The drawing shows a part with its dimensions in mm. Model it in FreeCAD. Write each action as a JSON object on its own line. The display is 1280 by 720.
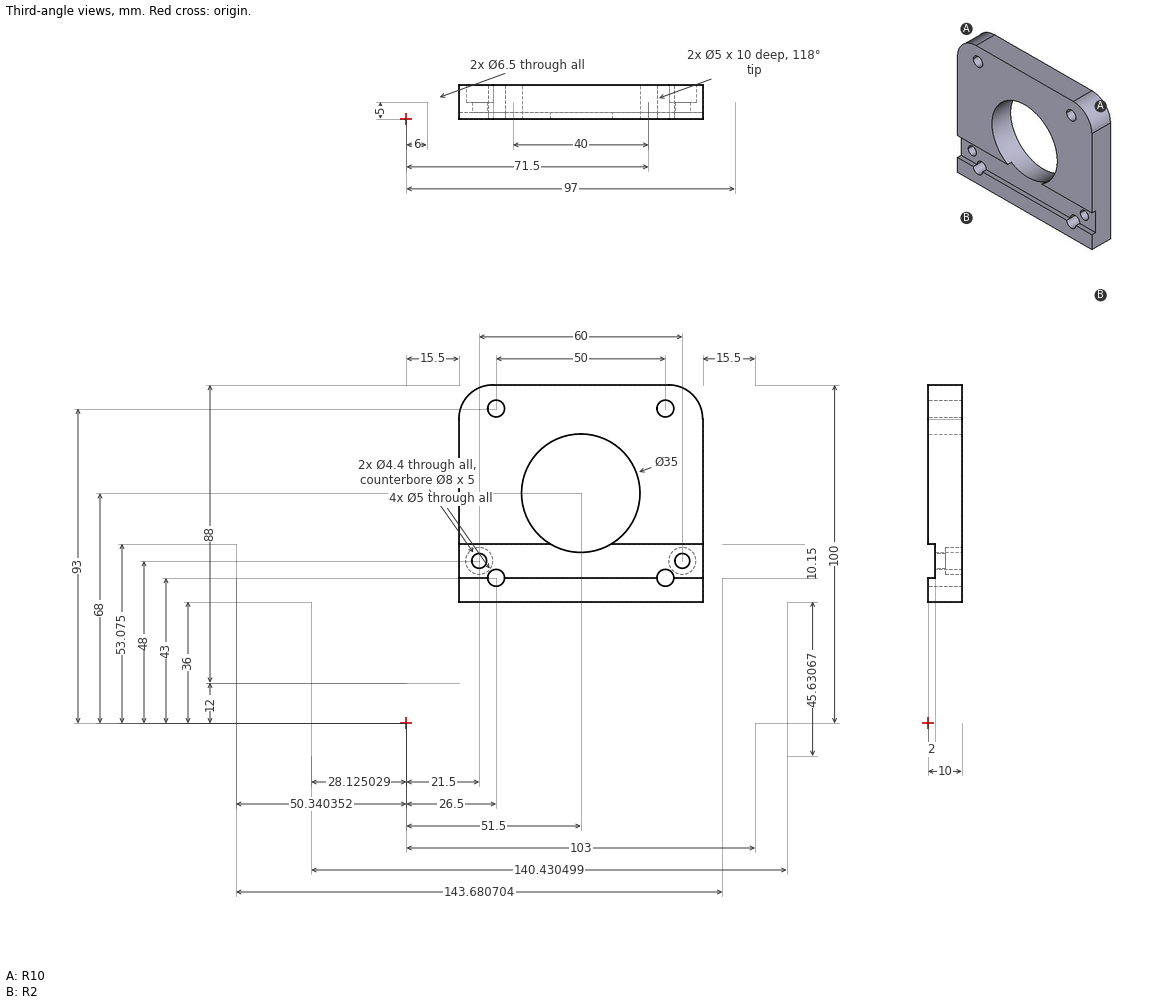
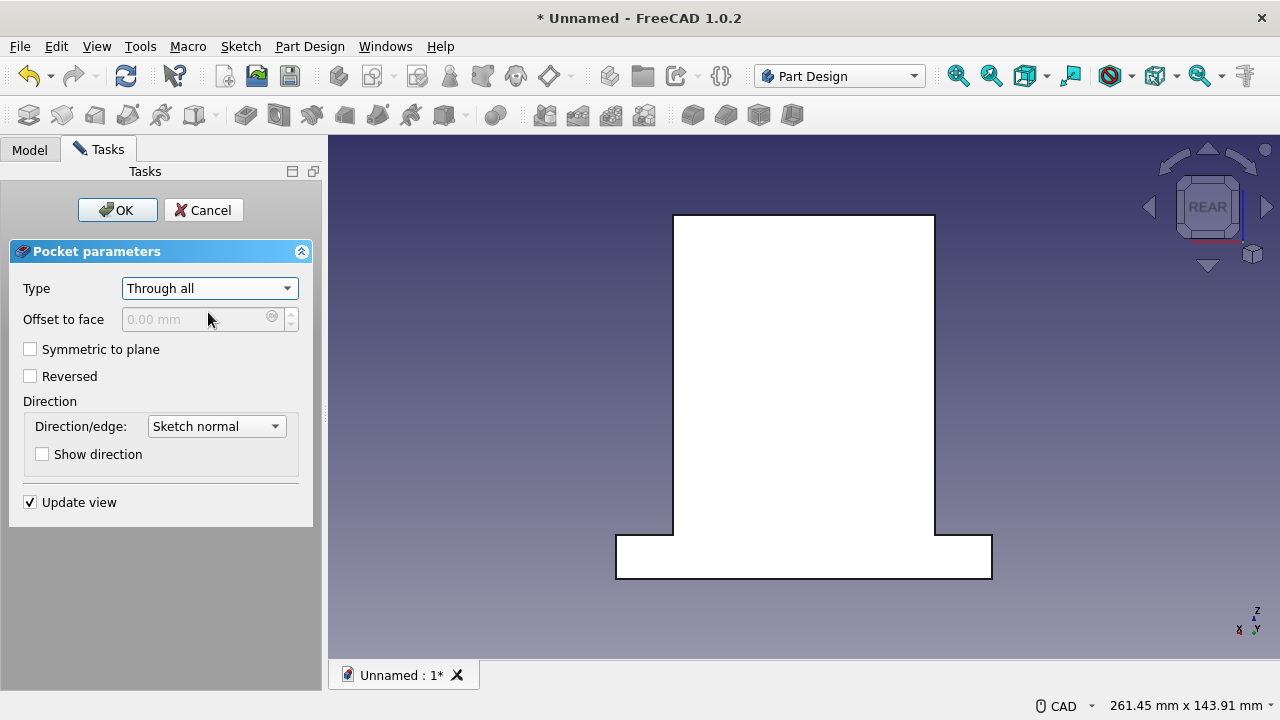
{"action": "left_click", "coordinate": [118, 210]}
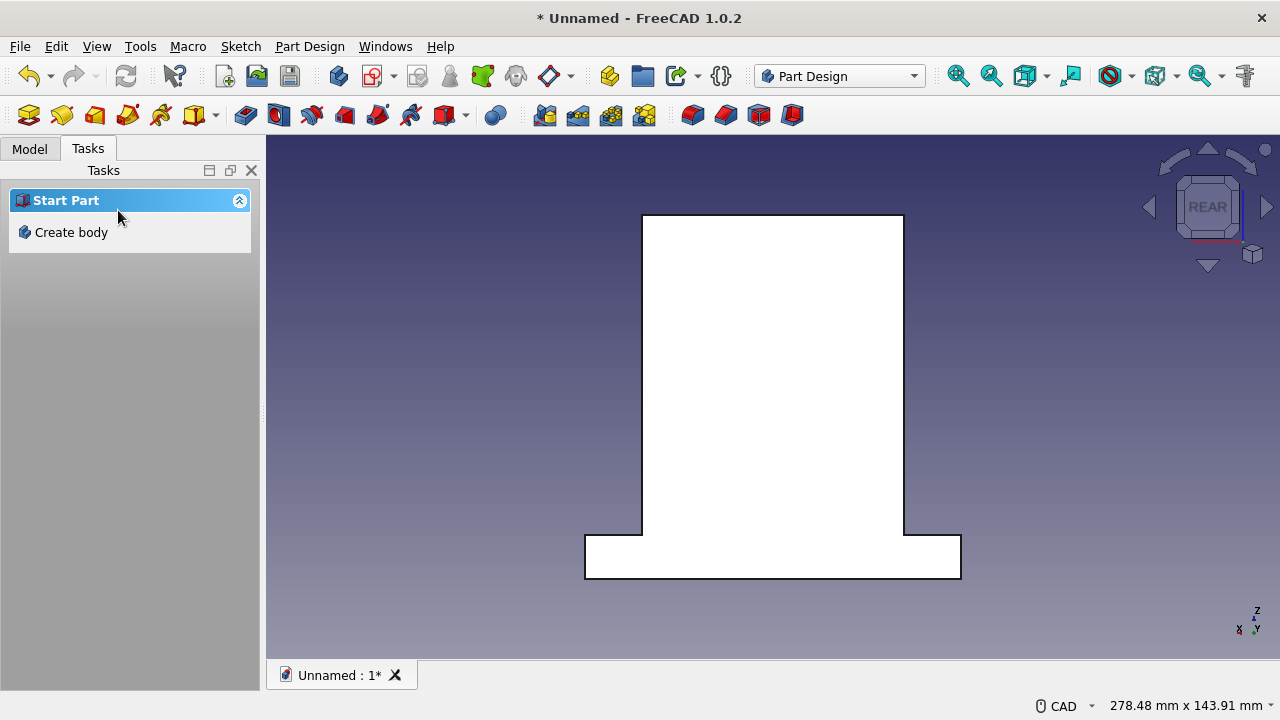
{"action": "key", "text": "0"}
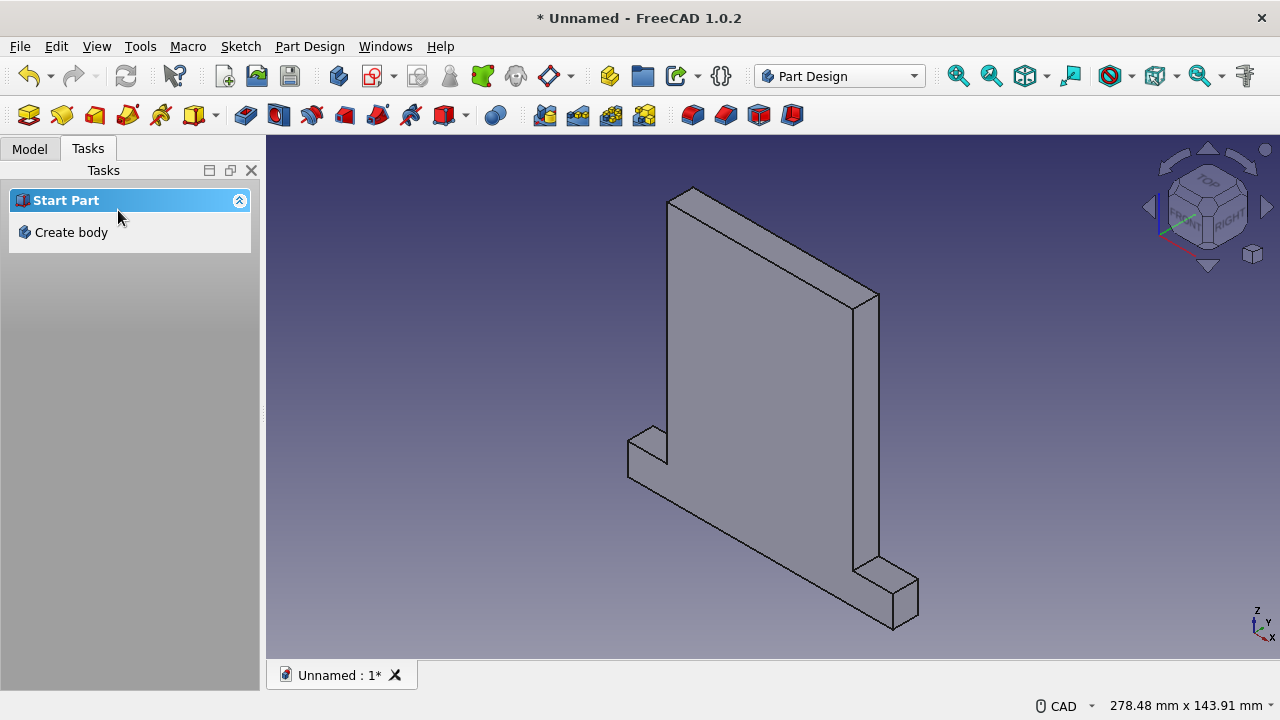
{"action": "left_click", "coordinate": [655, 441]}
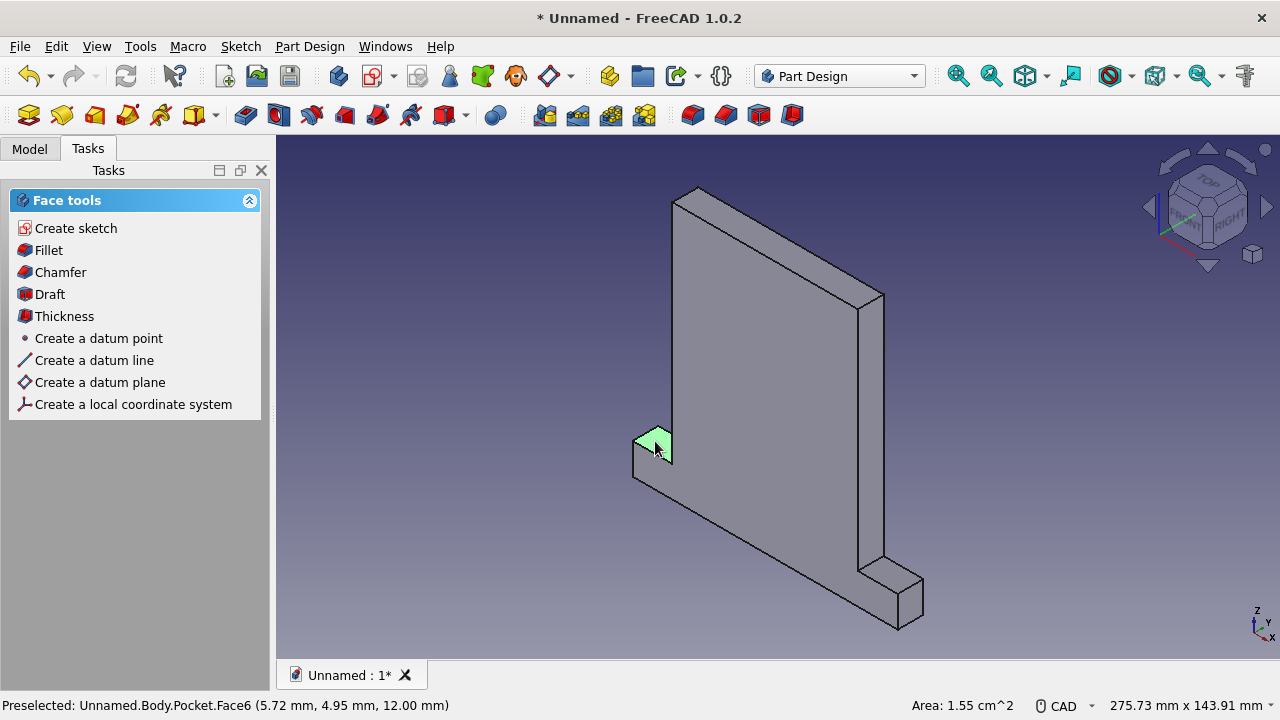
{"action": "left_click", "coordinate": [372, 76]}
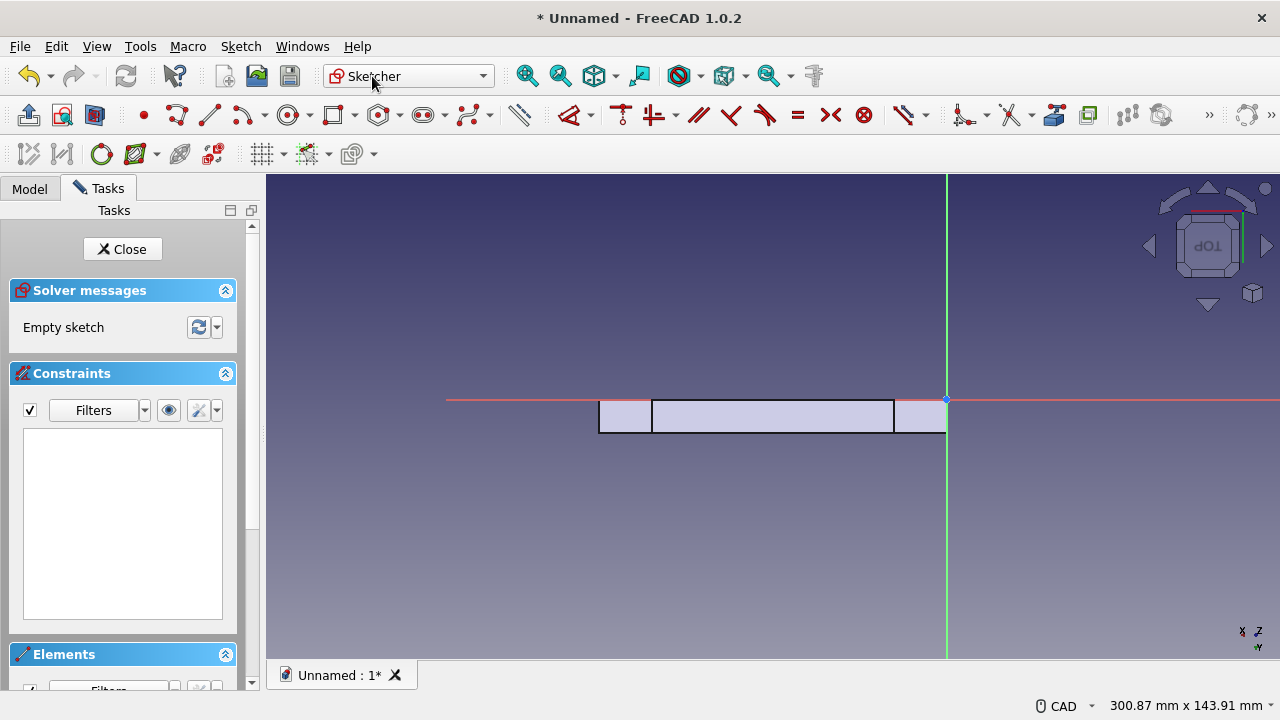
{"action": "scroll", "coordinate": [867, 410], "scroll_direction": "up", "scroll_amount": 3}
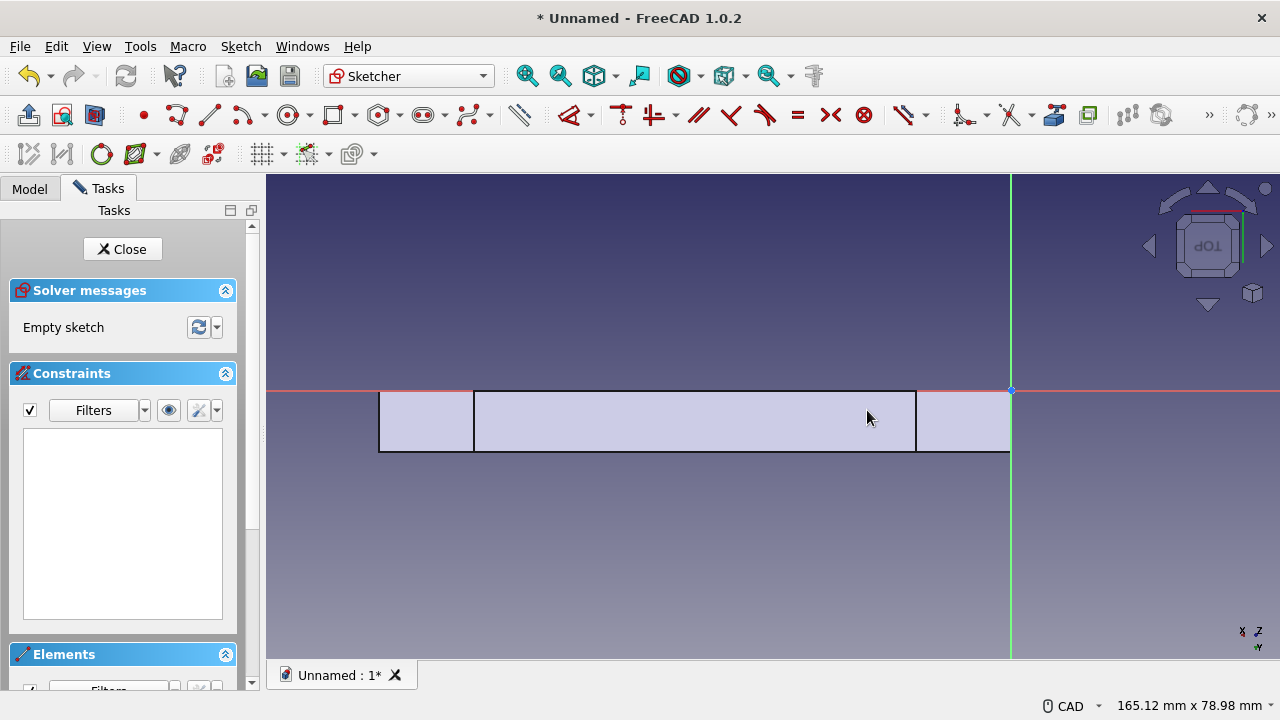
{"action": "left_click", "coordinate": [288, 116]}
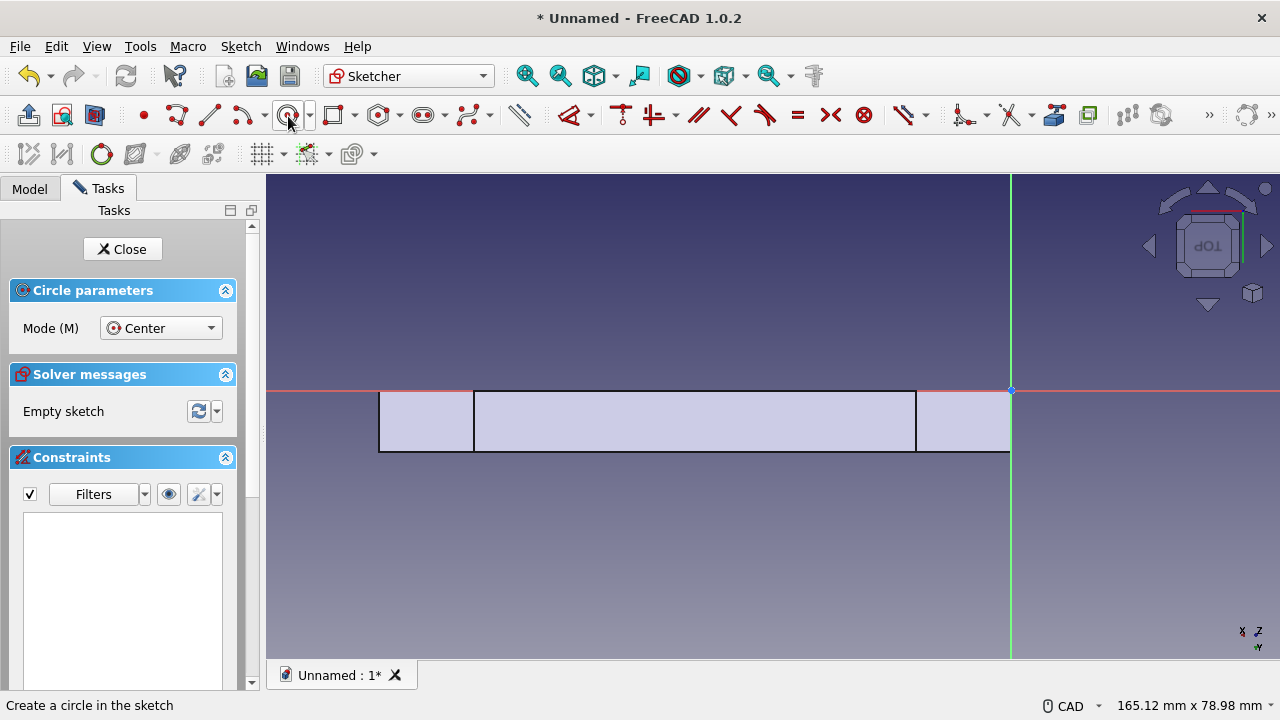
{"action": "left_click", "coordinate": [975, 421]}
{"action": "mouse_move", "coordinate": [989, 407]}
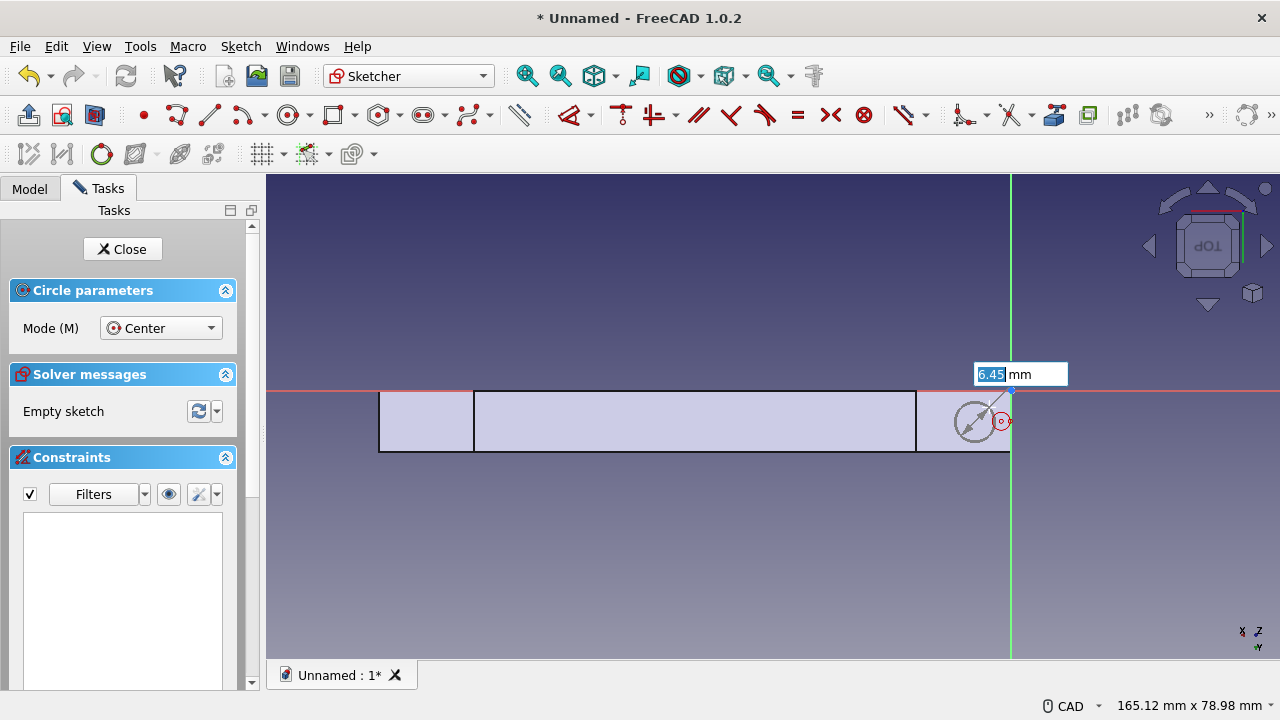
{"action": "type", "text": "6.5"}
{"action": "key", "text": "Return"}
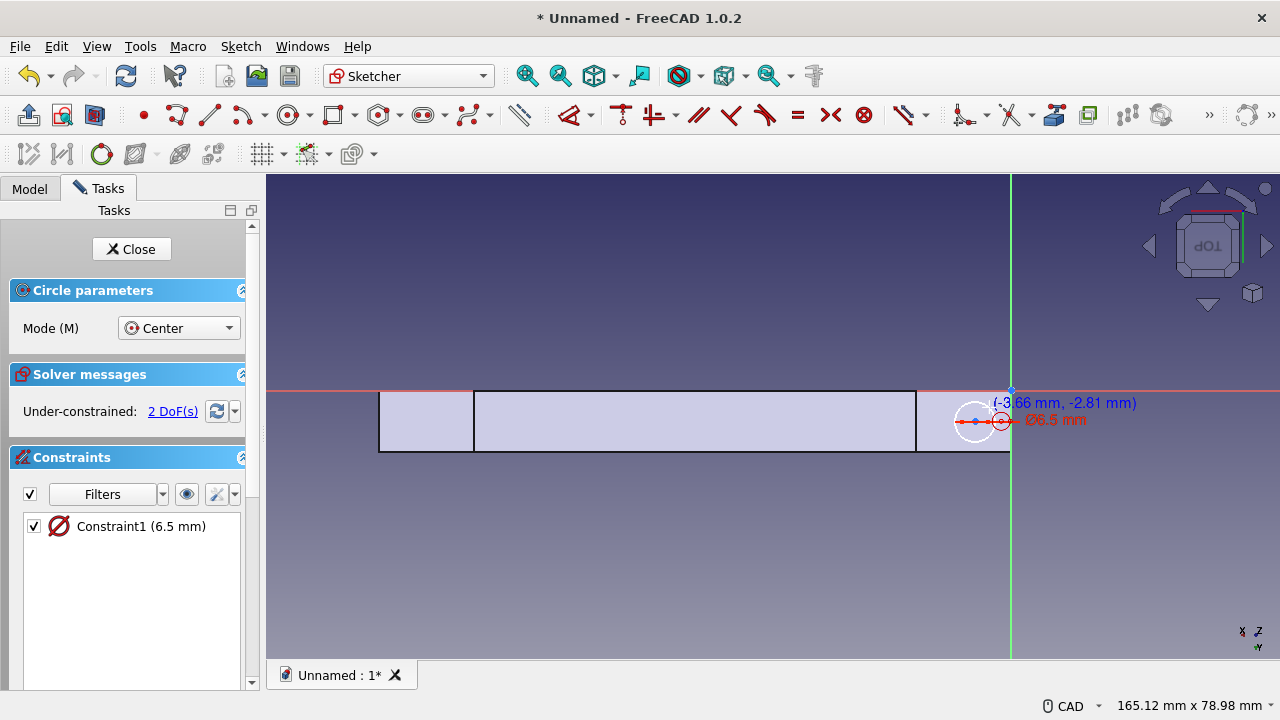
{"action": "left_click", "coordinate": [416, 421]}
{"action": "mouse_move", "coordinate": [430, 407]}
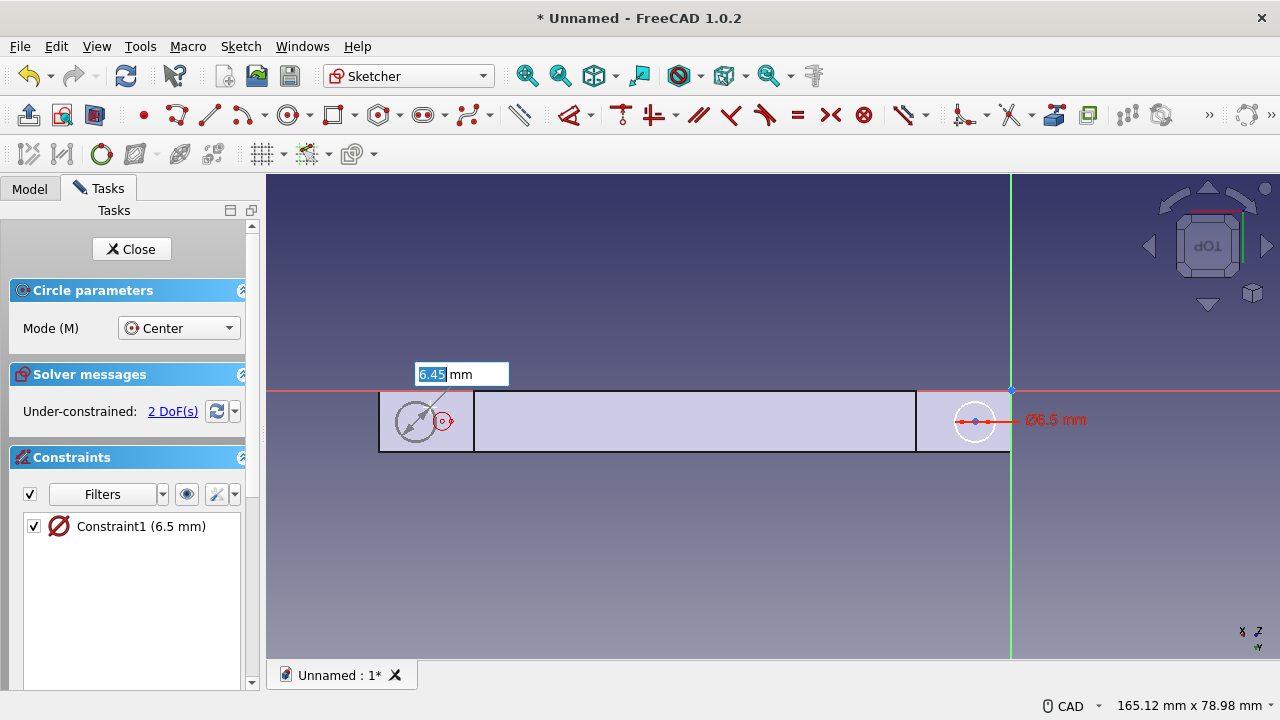
{"action": "type", "text": "6.5"}
{"action": "key", "text": "Return"}
{"action": "key", "text": "Escape"}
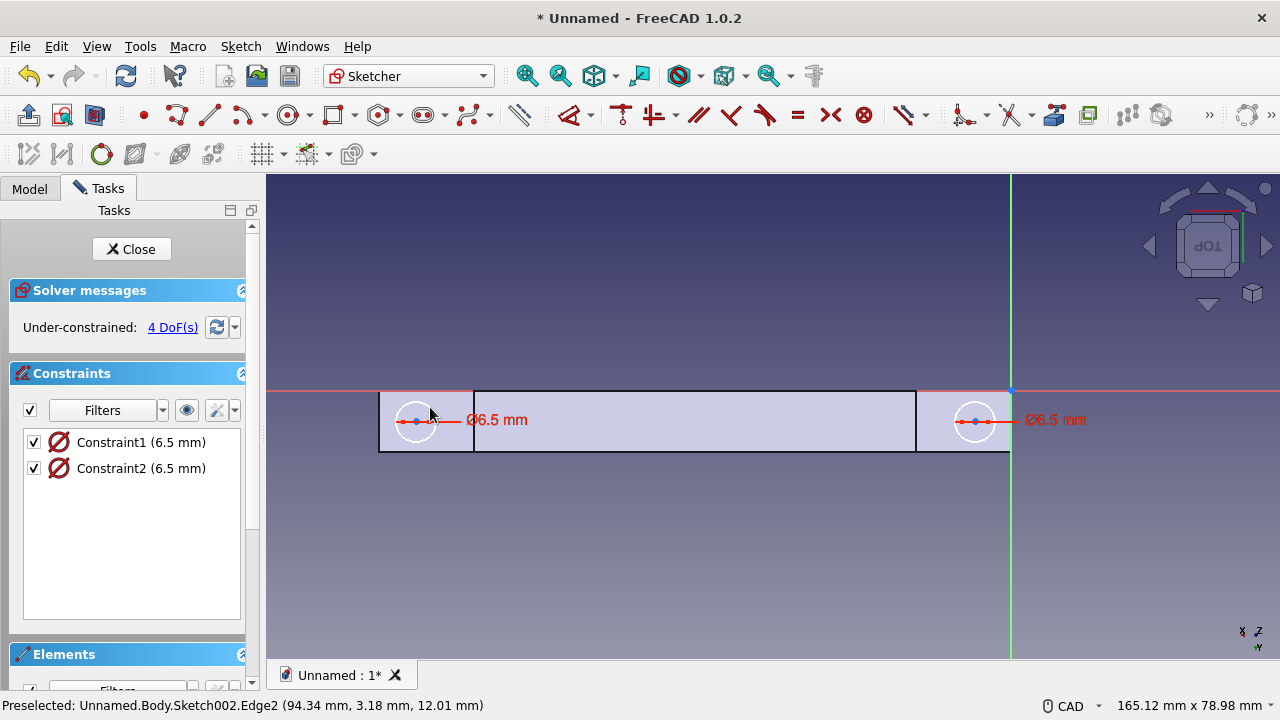
{"action": "key", "text": "d"}